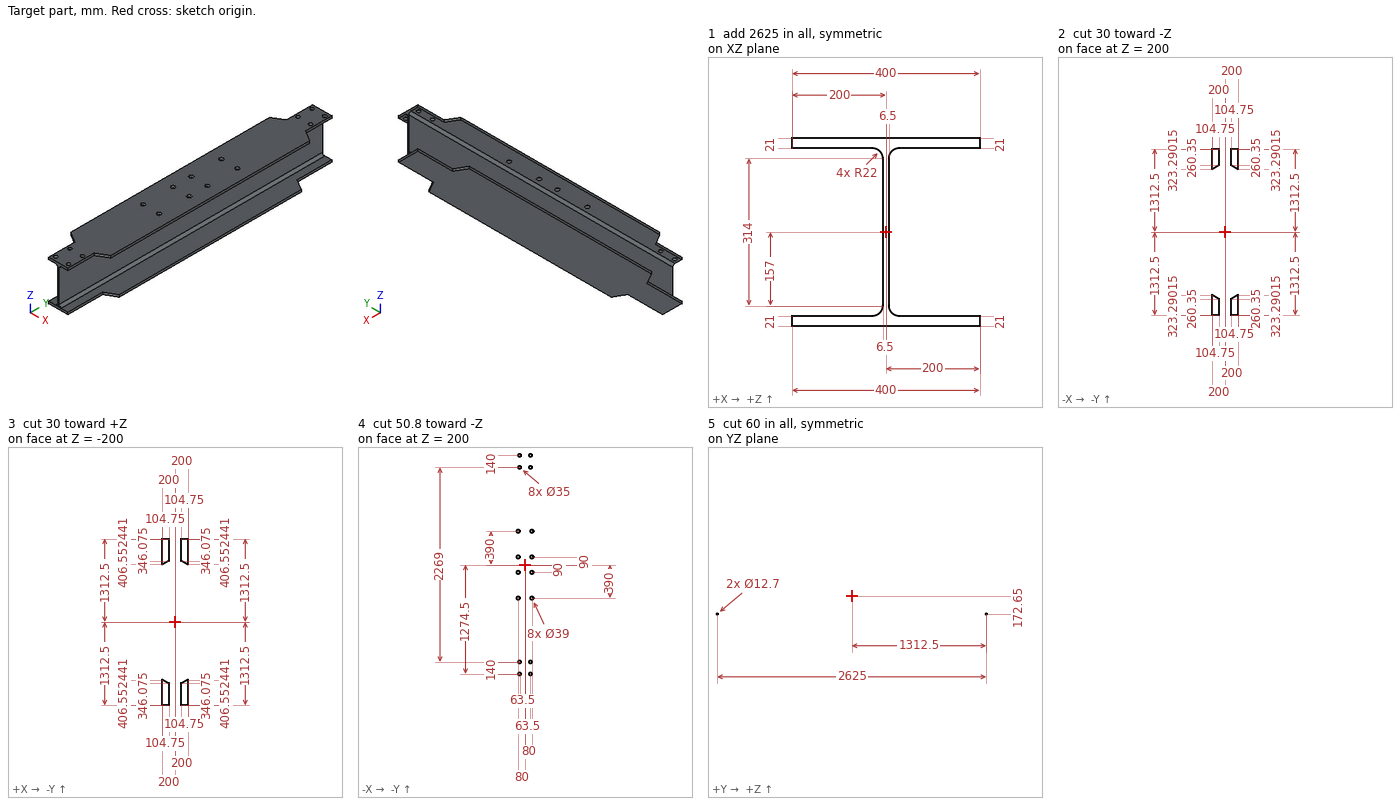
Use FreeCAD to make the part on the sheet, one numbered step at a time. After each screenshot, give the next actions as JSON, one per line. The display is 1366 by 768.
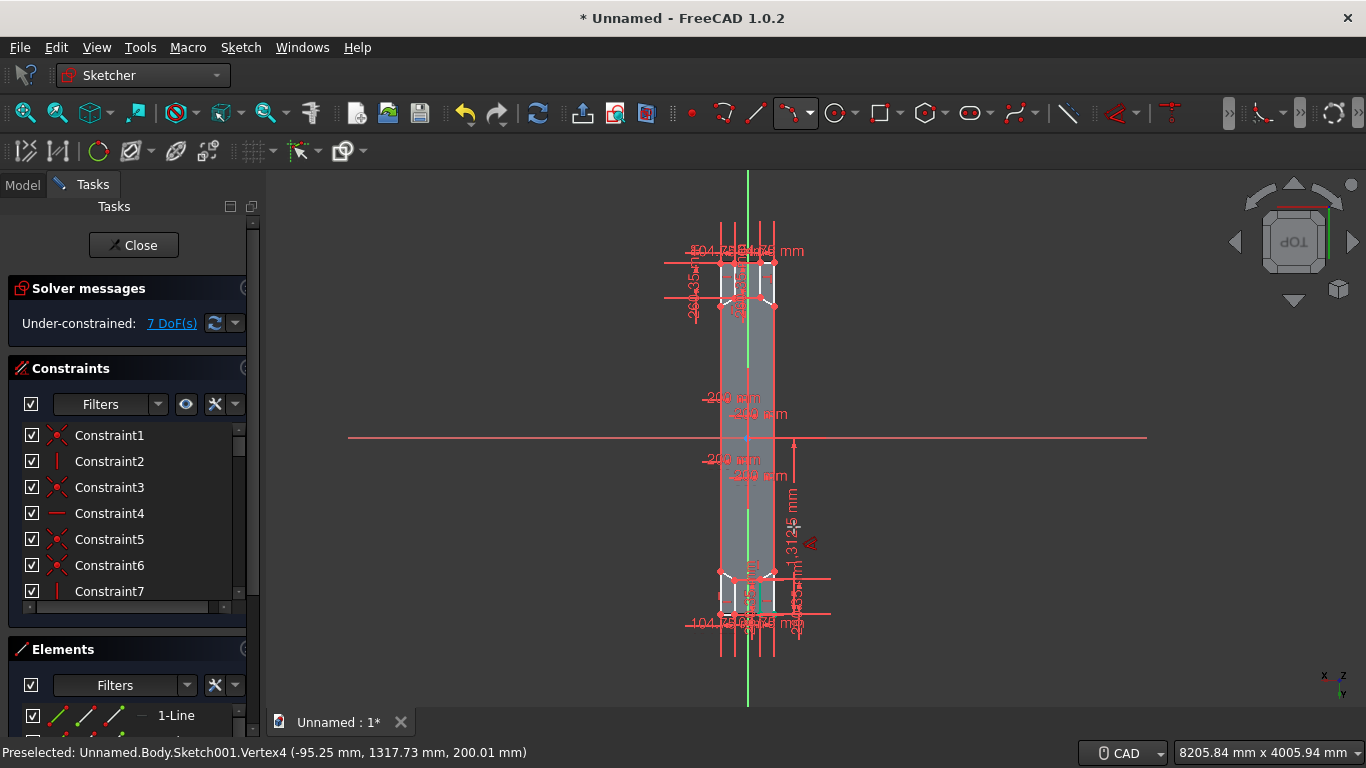
{"action": "left_click", "coordinate": [721, 615]}
{"action": "left_click", "coordinate": [687, 527]}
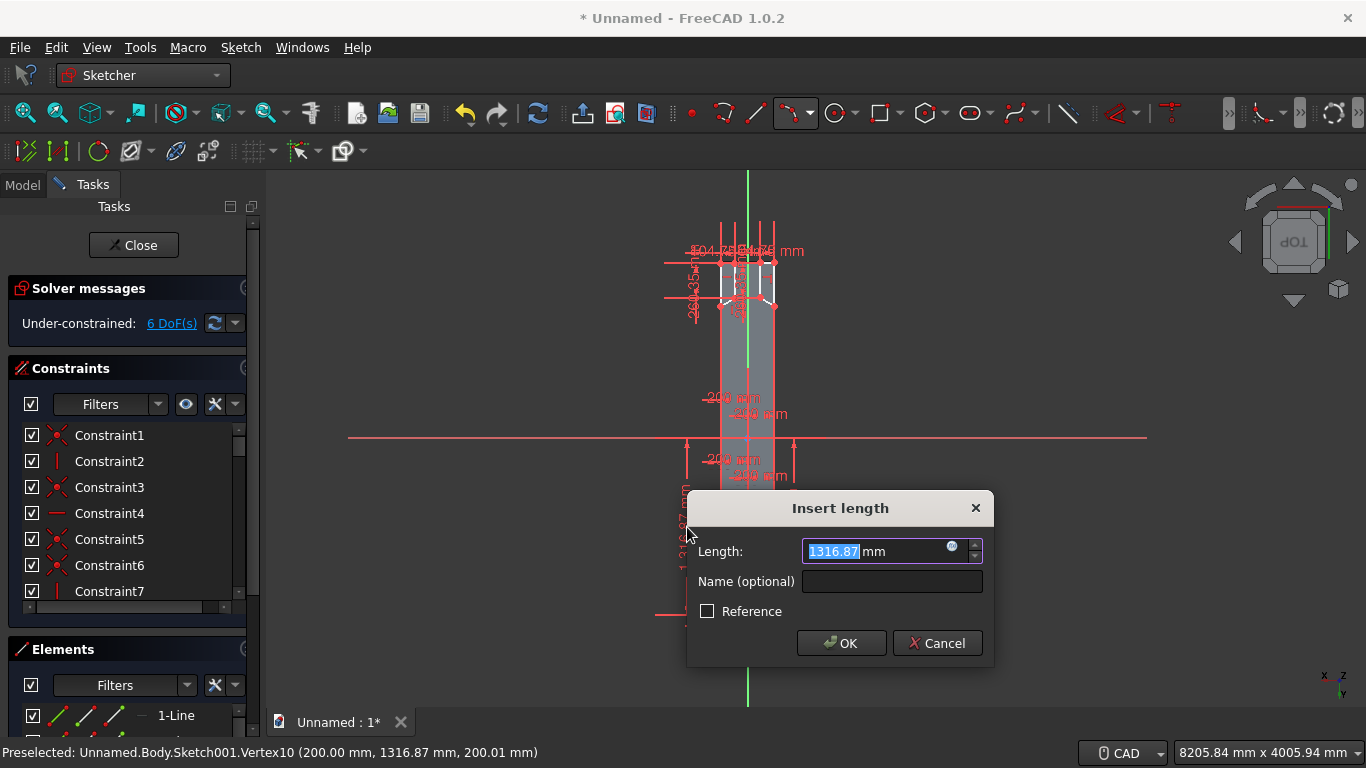
{"action": "type", "text": "1312.5"}
{"action": "key", "text": "Return"}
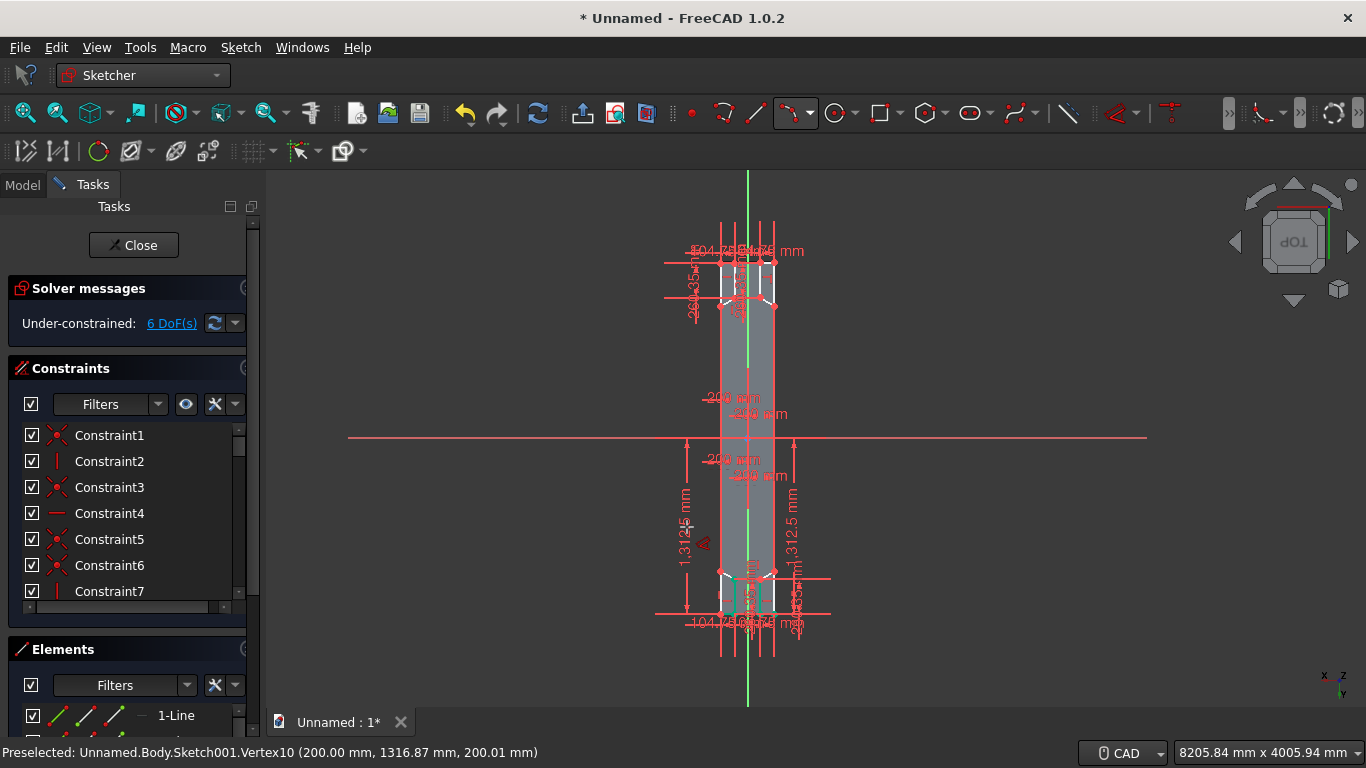
{"action": "left_click", "coordinate": [735, 263]}
{"action": "left_click", "coordinate": [701, 351]}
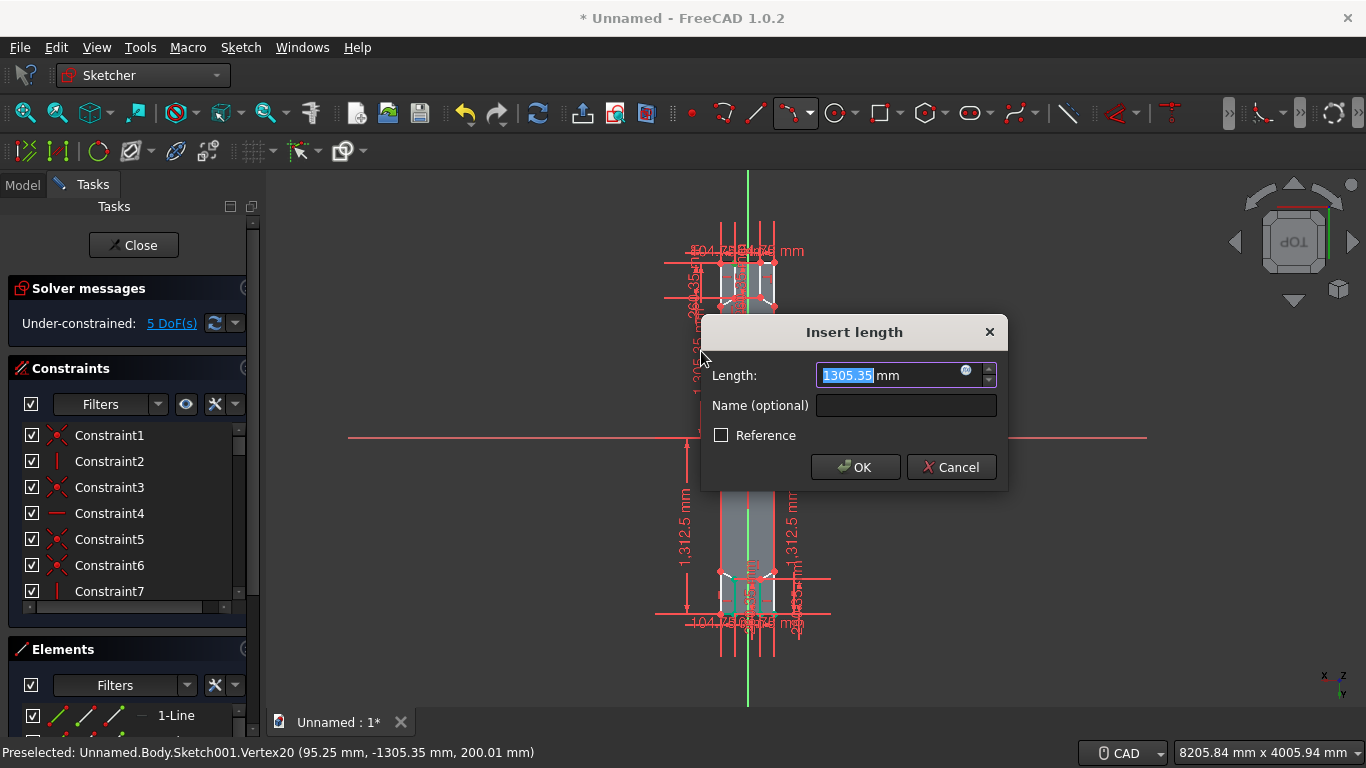
{"action": "type", "text": "1312.5"}
{"action": "key", "text": "Return"}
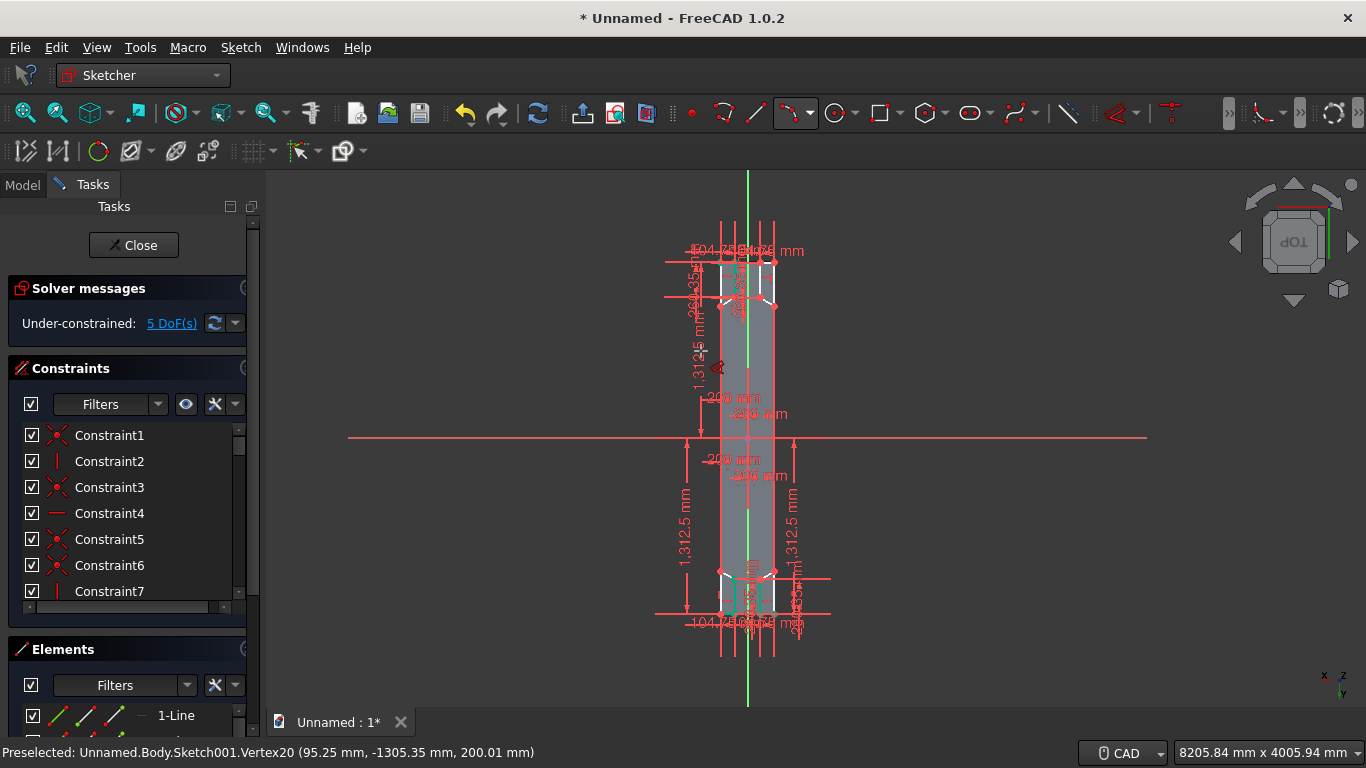
{"action": "left_click", "coordinate": [774, 263]}
{"action": "left_click", "coordinate": [808, 351]}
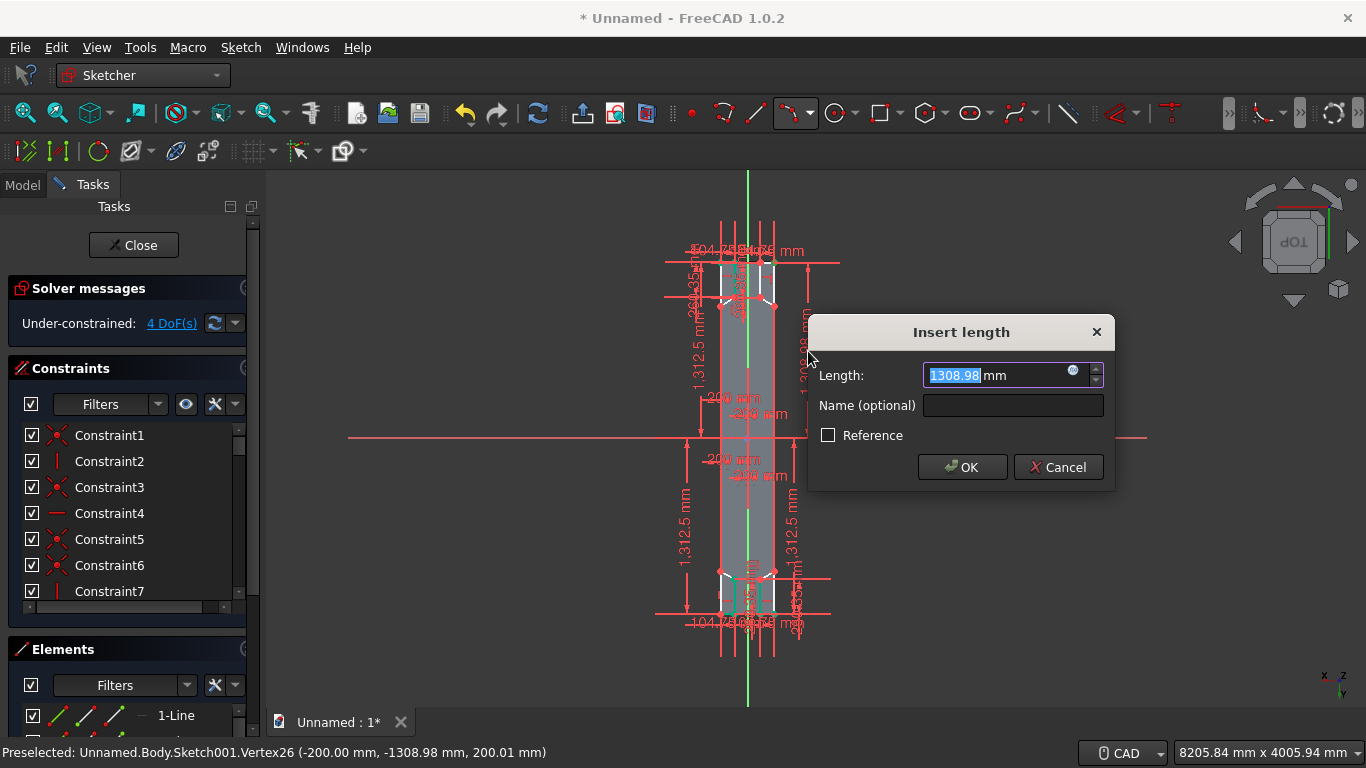
{"action": "type", "text": "1312.5"}
{"action": "key", "text": "Return"}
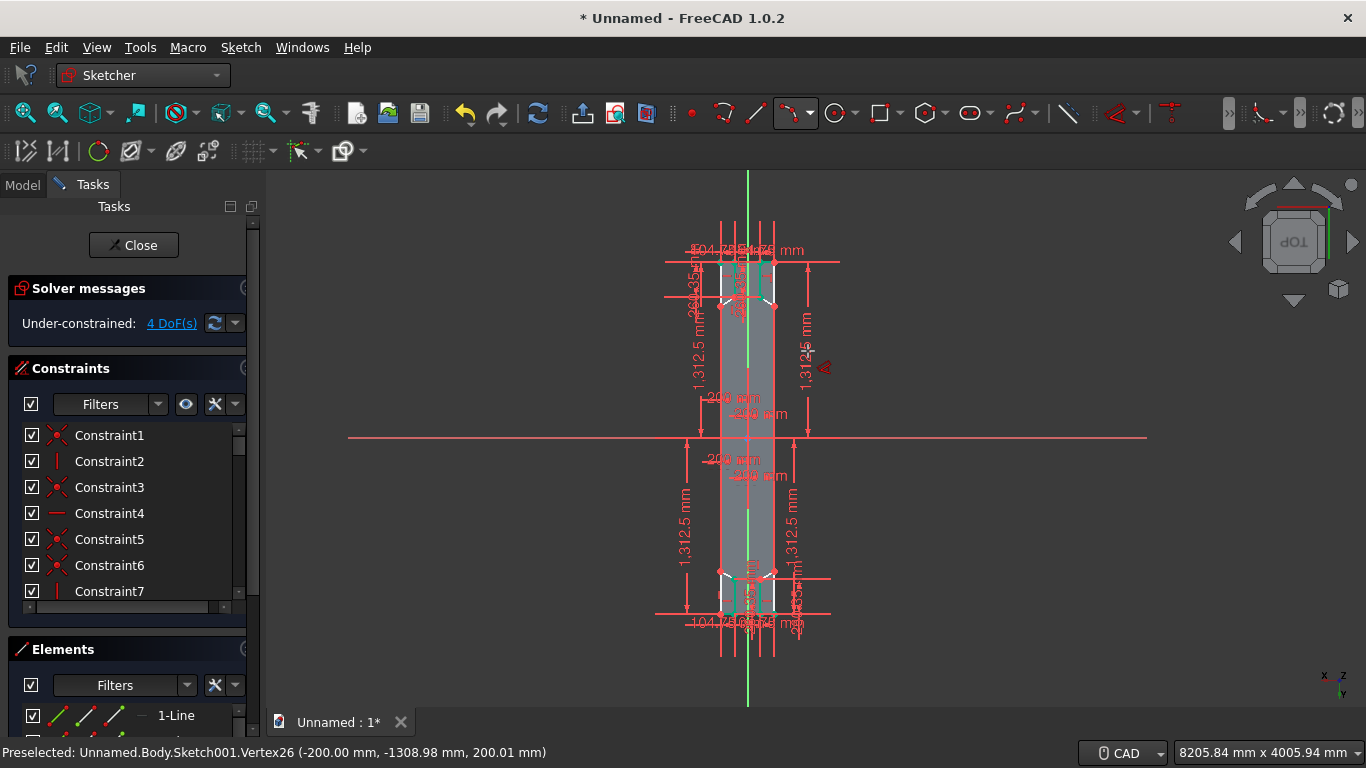
{"action": "left_click", "coordinate": [774, 602]}
{"action": "left_click", "coordinate": [880, 593]}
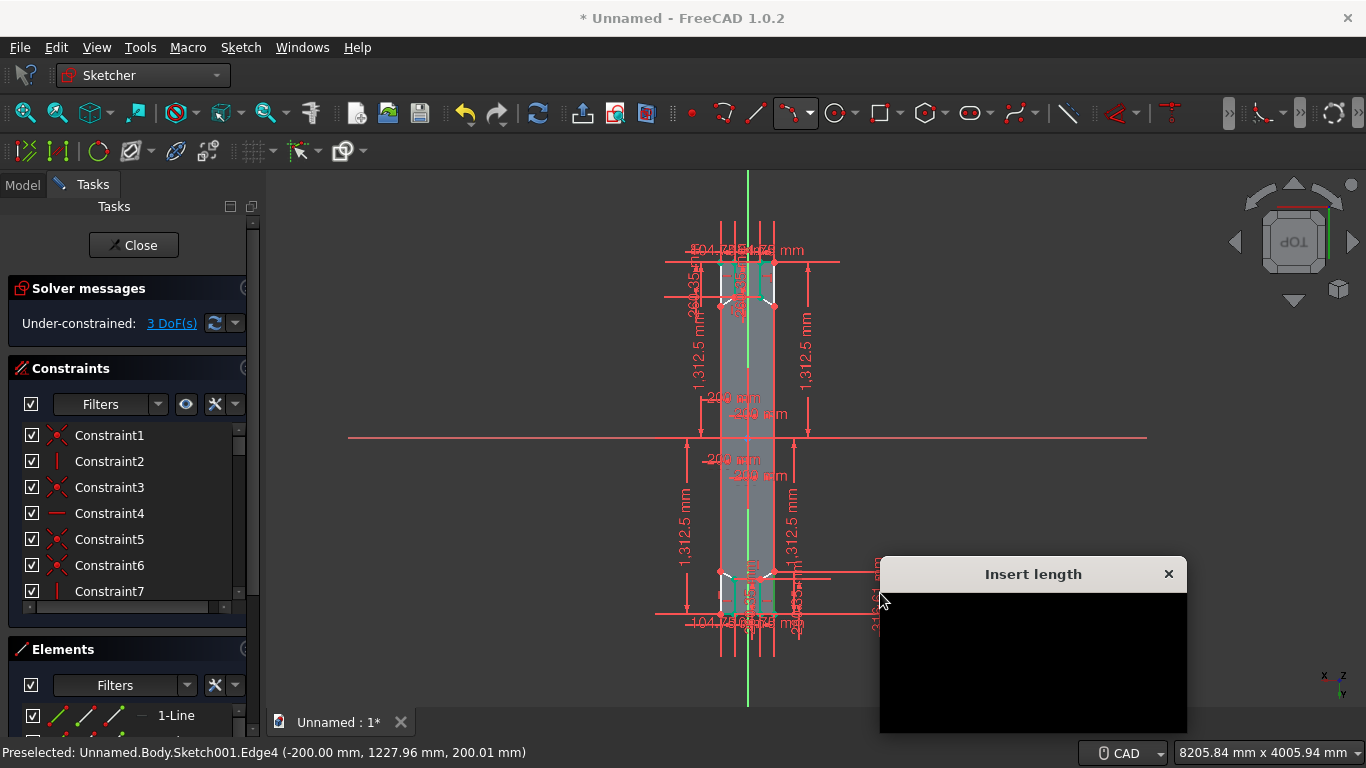
{"action": "type", "text": "323.29015"}
{"action": "key", "text": "Return"}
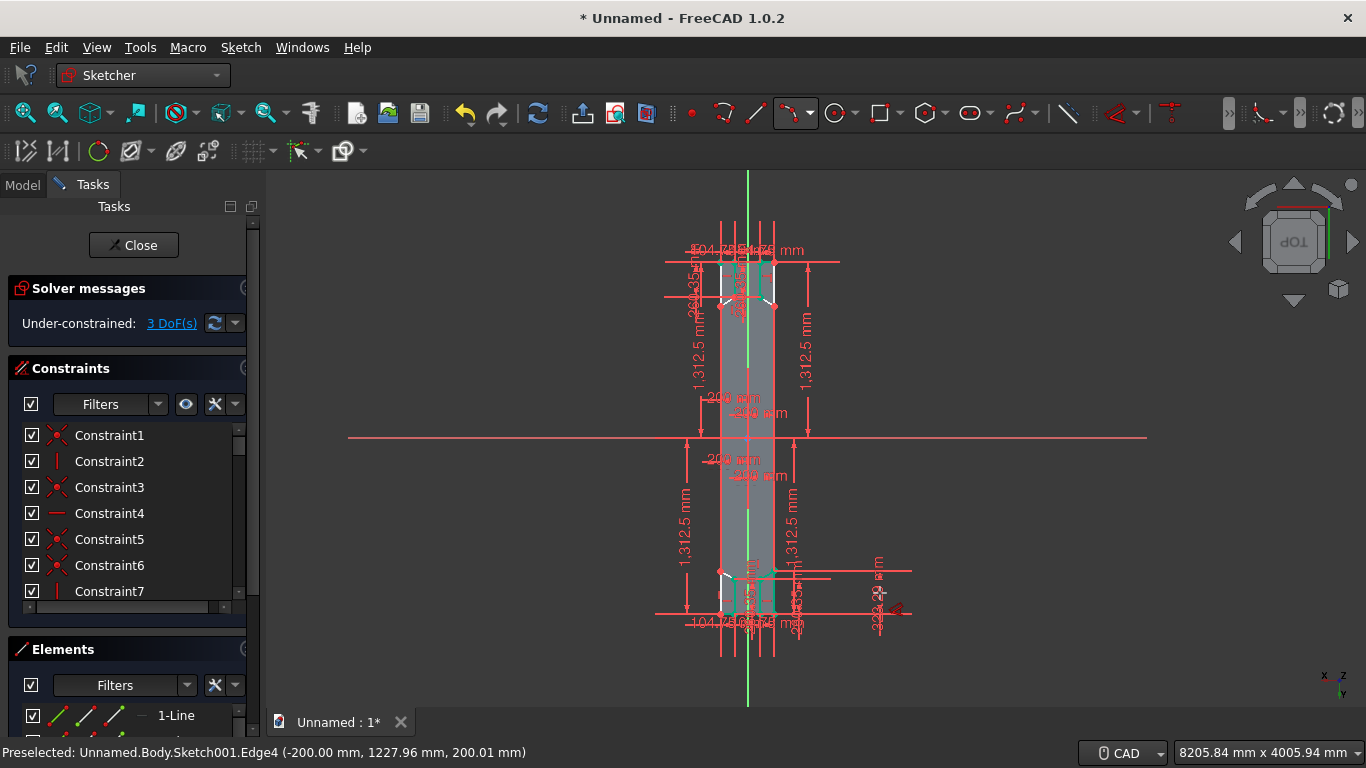
{"action": "scroll", "coordinate": [721, 584], "scroll_direction": "up", "scroll_amount": 2}